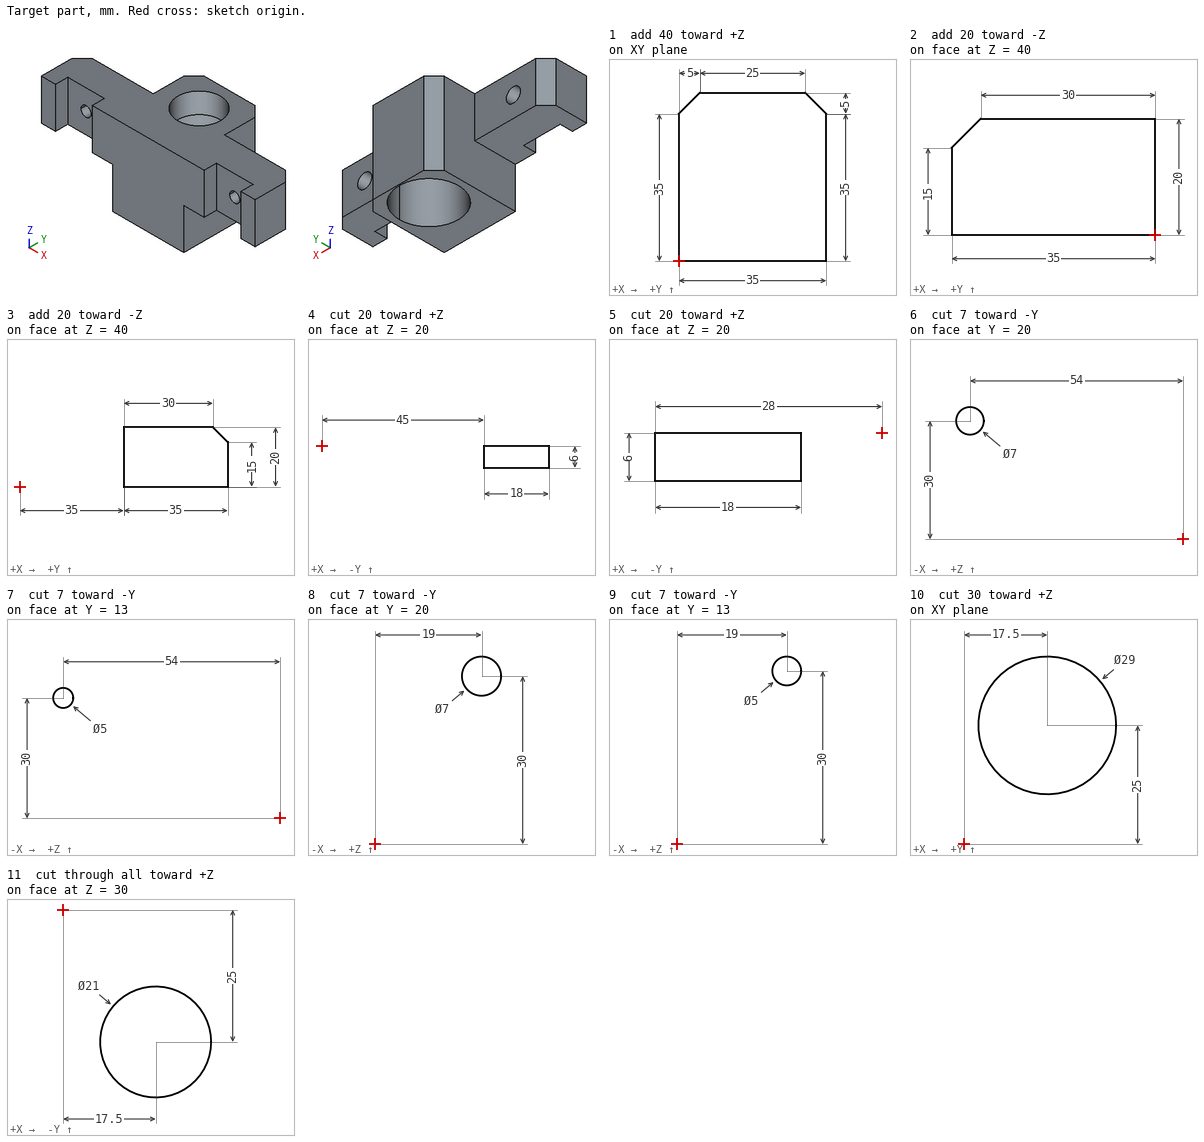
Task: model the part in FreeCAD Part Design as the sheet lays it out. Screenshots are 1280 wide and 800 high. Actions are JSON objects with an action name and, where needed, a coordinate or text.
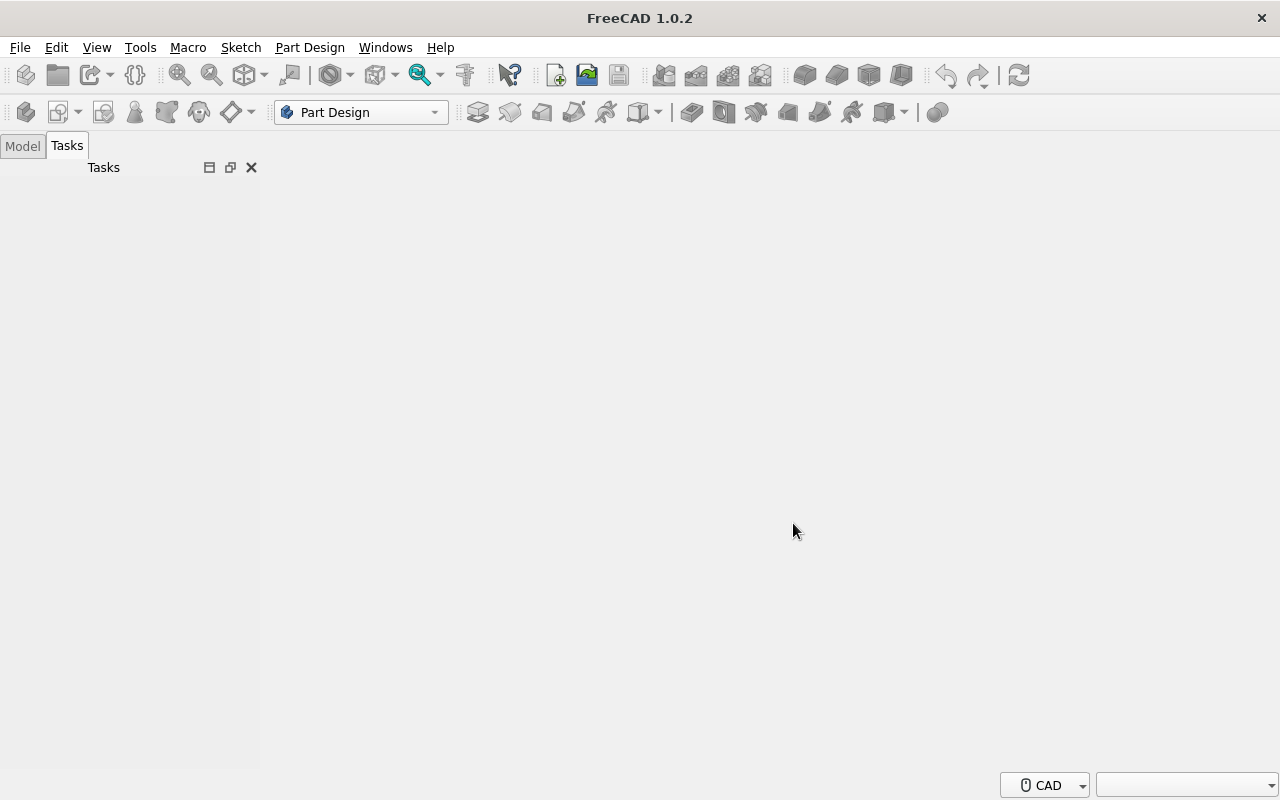
{"action": "left_click", "coordinate": [556, 76]}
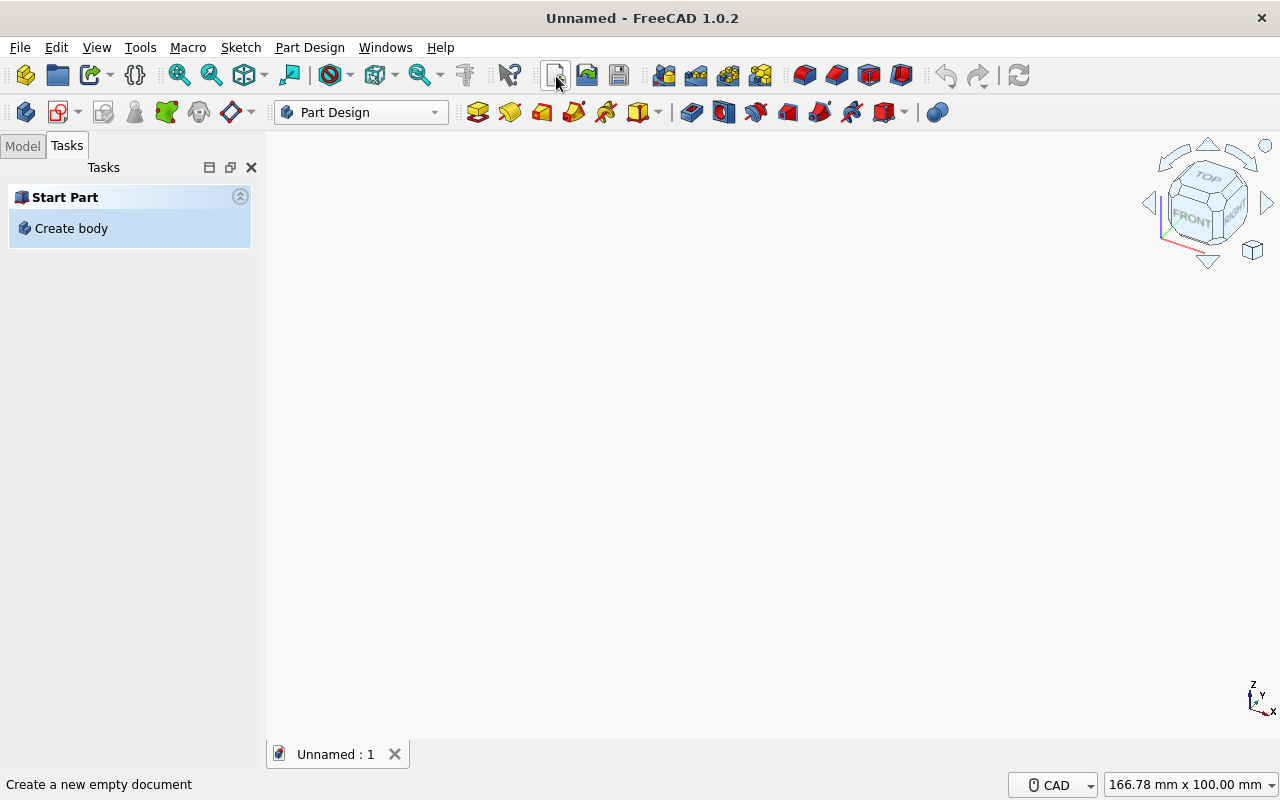
{"action": "left_click", "coordinate": [58, 112]}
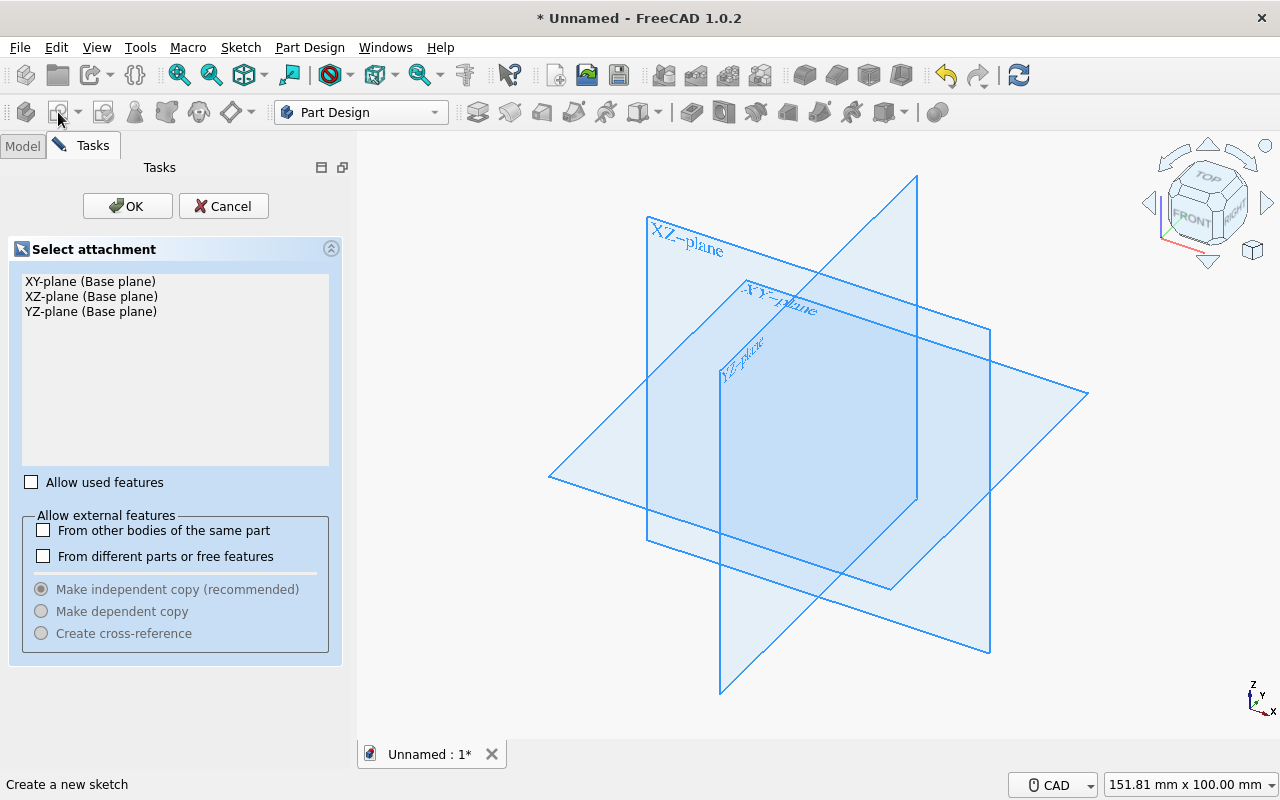
{"action": "left_click", "coordinate": [82, 282]}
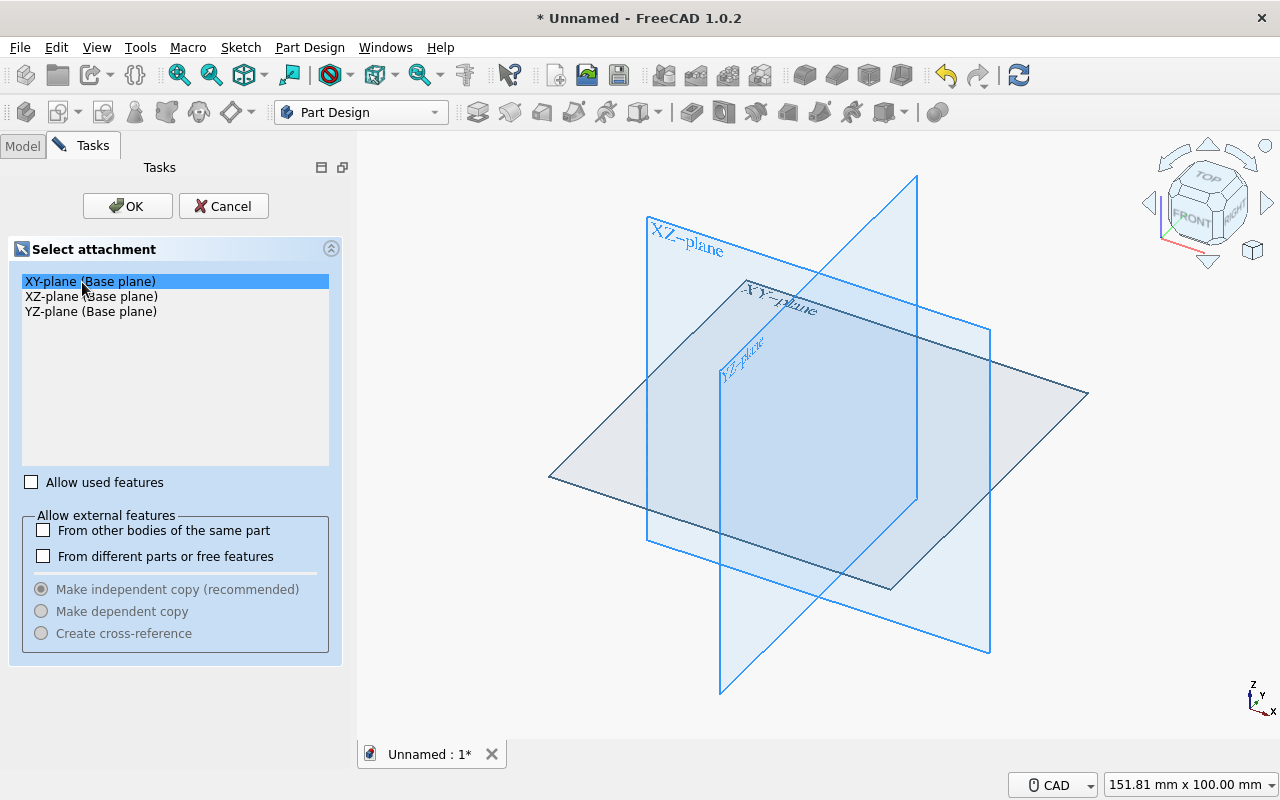
{"action": "left_click", "coordinate": [128, 206]}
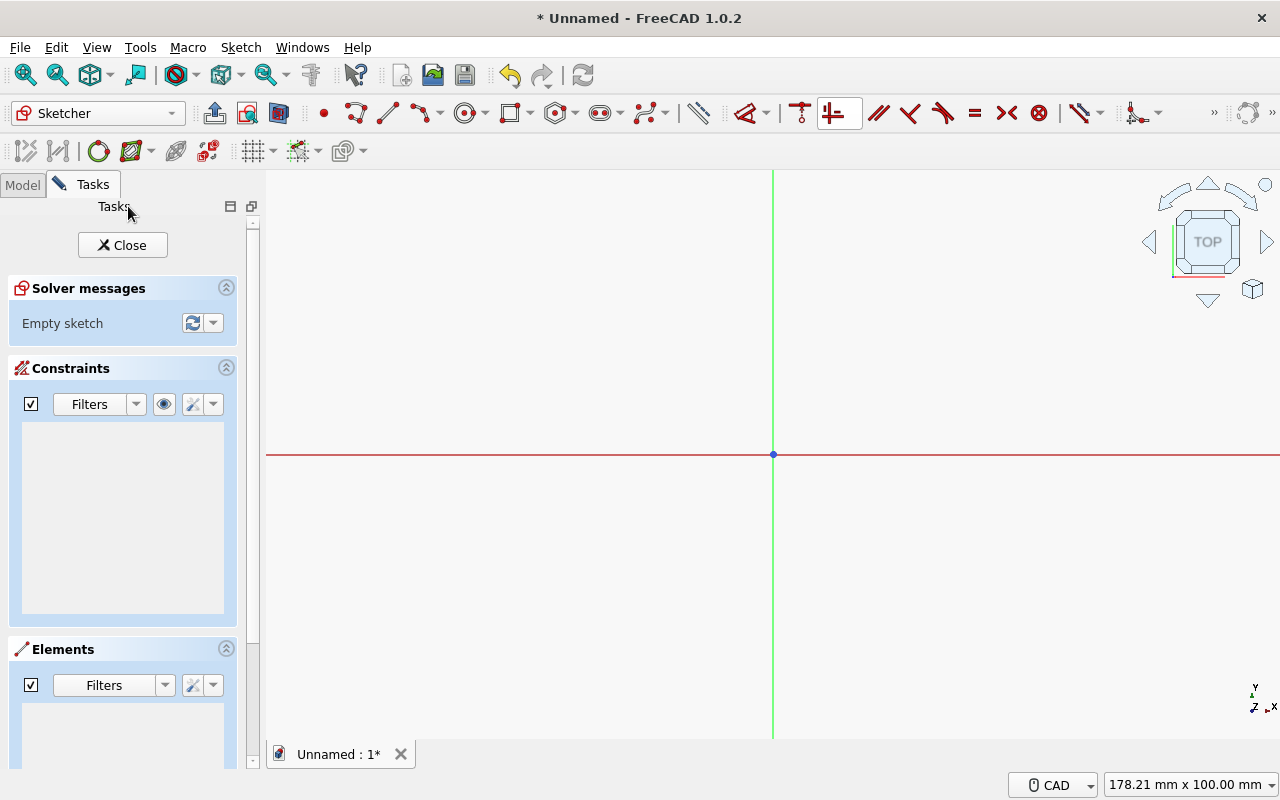
{"action": "scroll", "coordinate": [1115, 198], "scroll_direction": "up", "scroll_amount": 2}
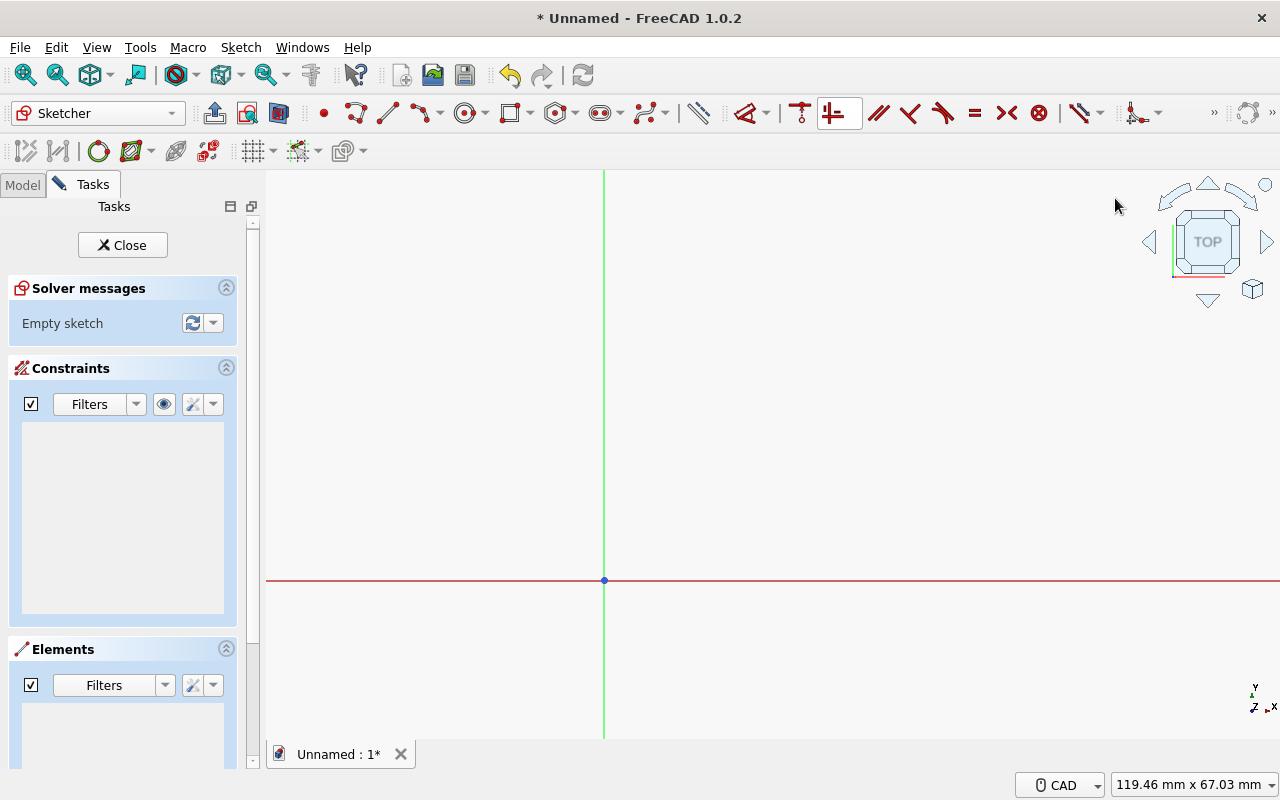
{"action": "left_click", "coordinate": [356, 114]}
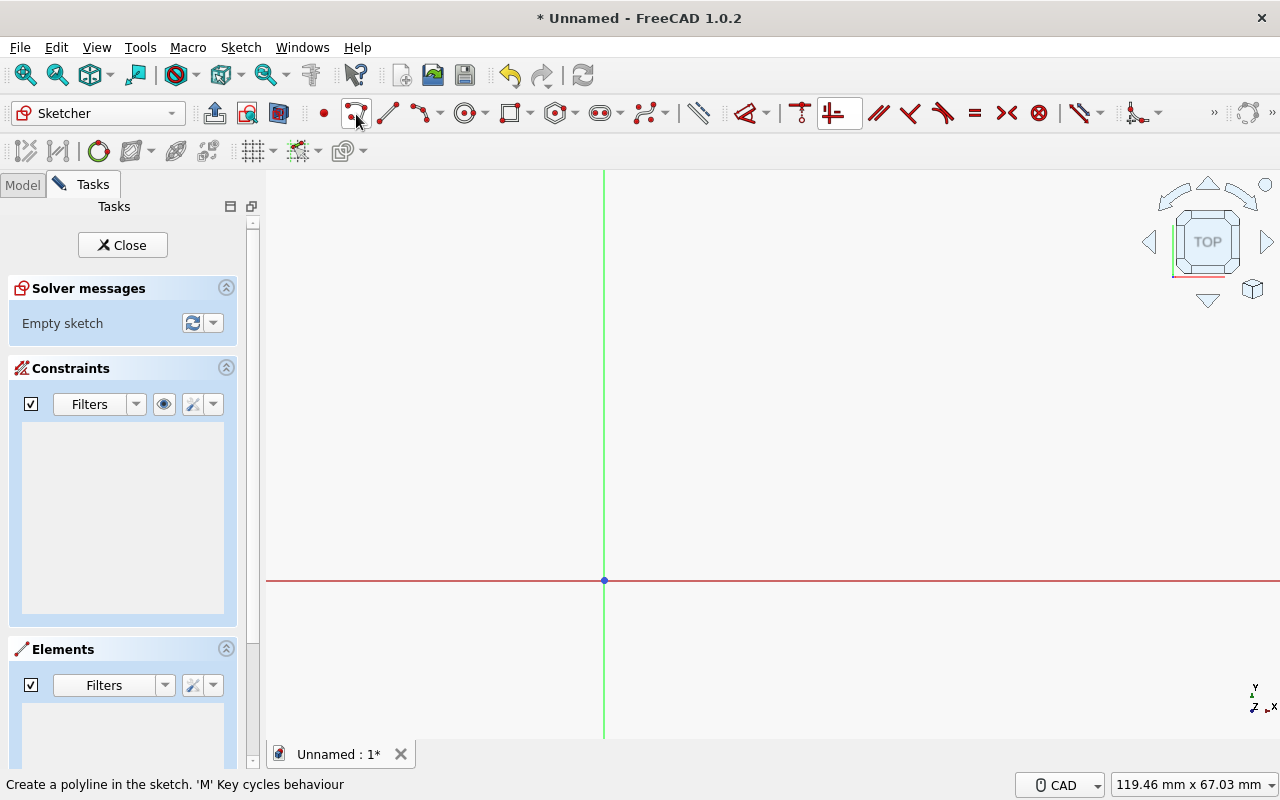
{"action": "left_click", "coordinate": [604, 581]}
{"action": "left_click", "coordinate": [901, 572]}
{"action": "left_click", "coordinate": [901, 284]}
{"action": "left_click", "coordinate": [859, 241]}
{"action": "left_click", "coordinate": [647, 241]}
{"action": "left_click", "coordinate": [613, 284]}
{"action": "left_click", "coordinate": [604, 581]}
{"action": "key", "text": "Escape"}
{"action": "key", "text": "Escape"}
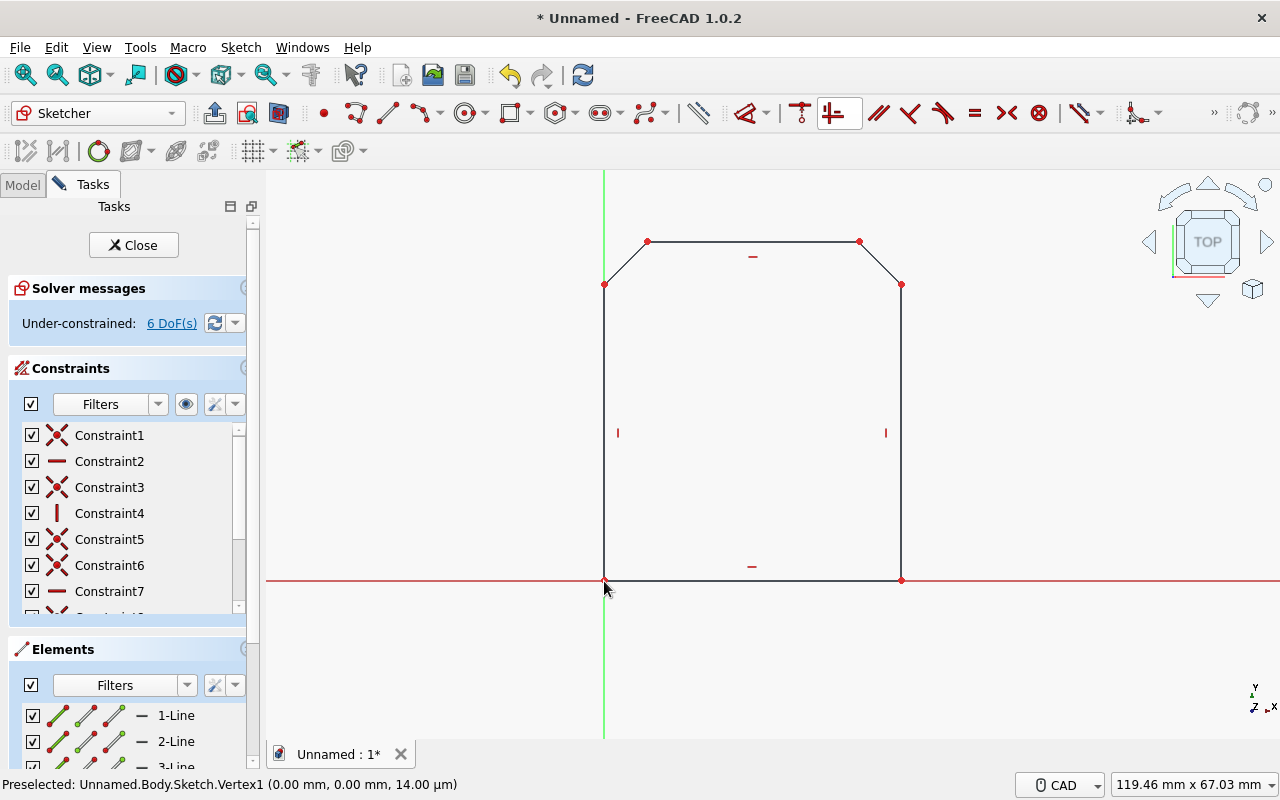
{"action": "left_click", "coordinate": [746, 114]}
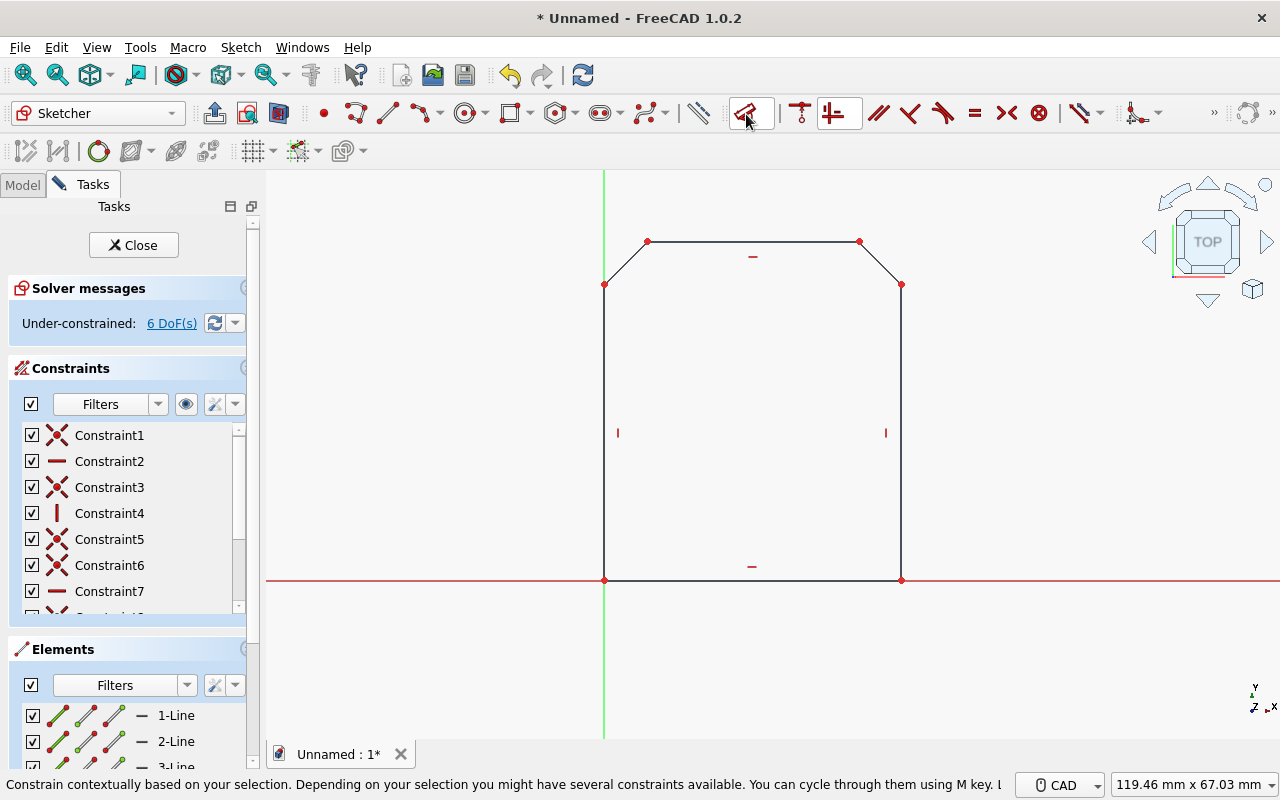
{"action": "left_click", "coordinate": [693, 581]}
{"action": "left_click", "coordinate": [753, 615]}